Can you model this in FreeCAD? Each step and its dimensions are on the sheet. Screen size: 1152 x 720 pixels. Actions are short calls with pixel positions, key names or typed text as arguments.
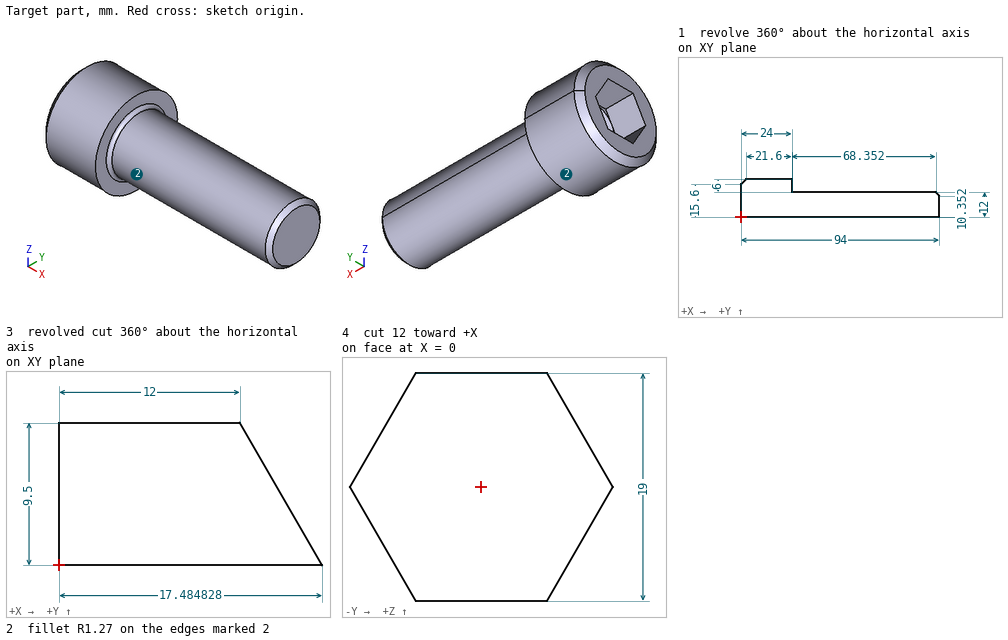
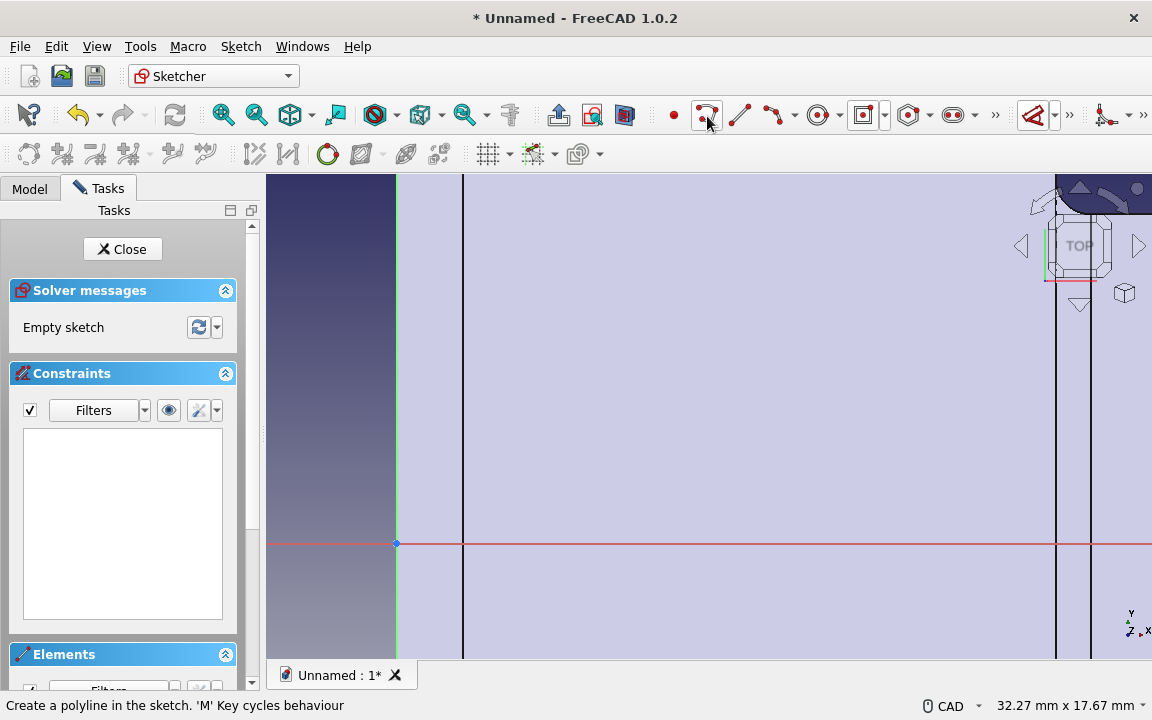
click(397, 544)
click(877, 535)
click(726, 283)
click(406, 283)
click(397, 544)
key(Escape)
key(Escape)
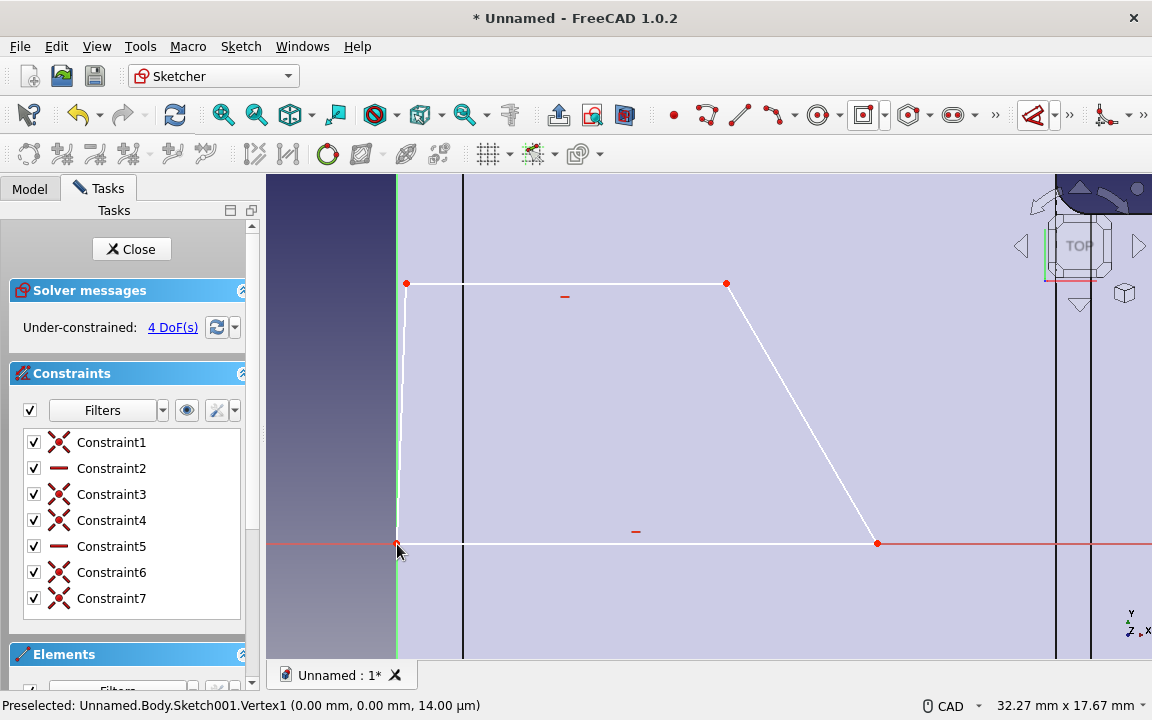
click(400, 466)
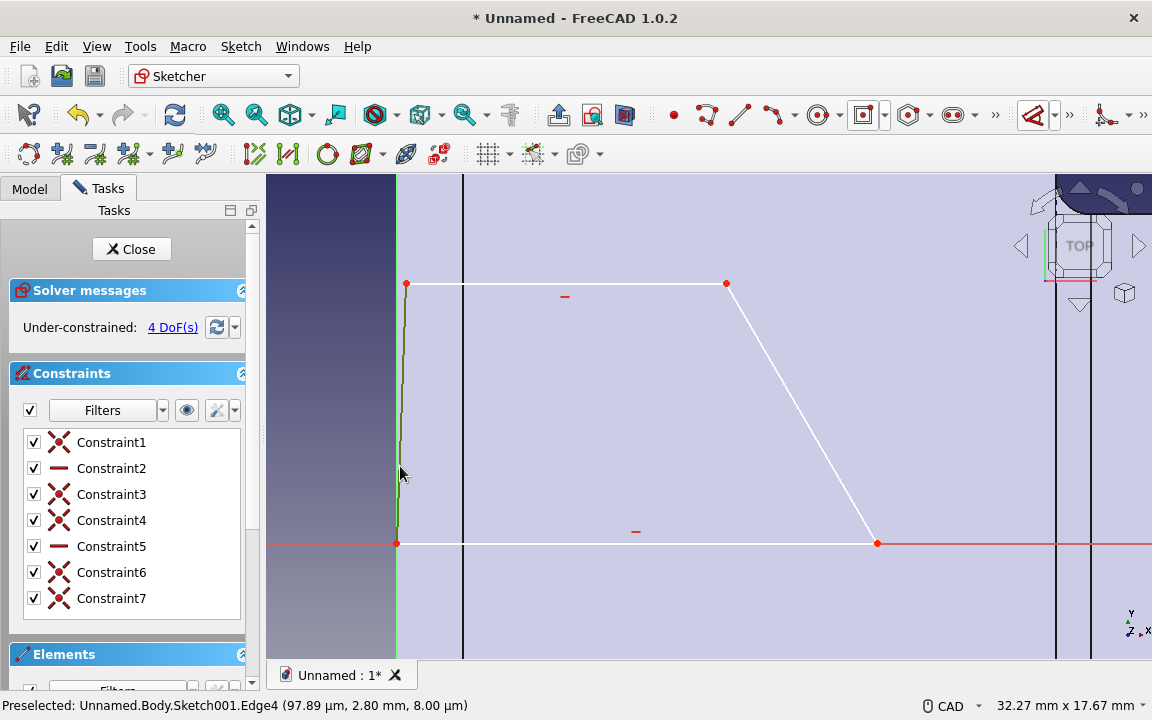
key(v)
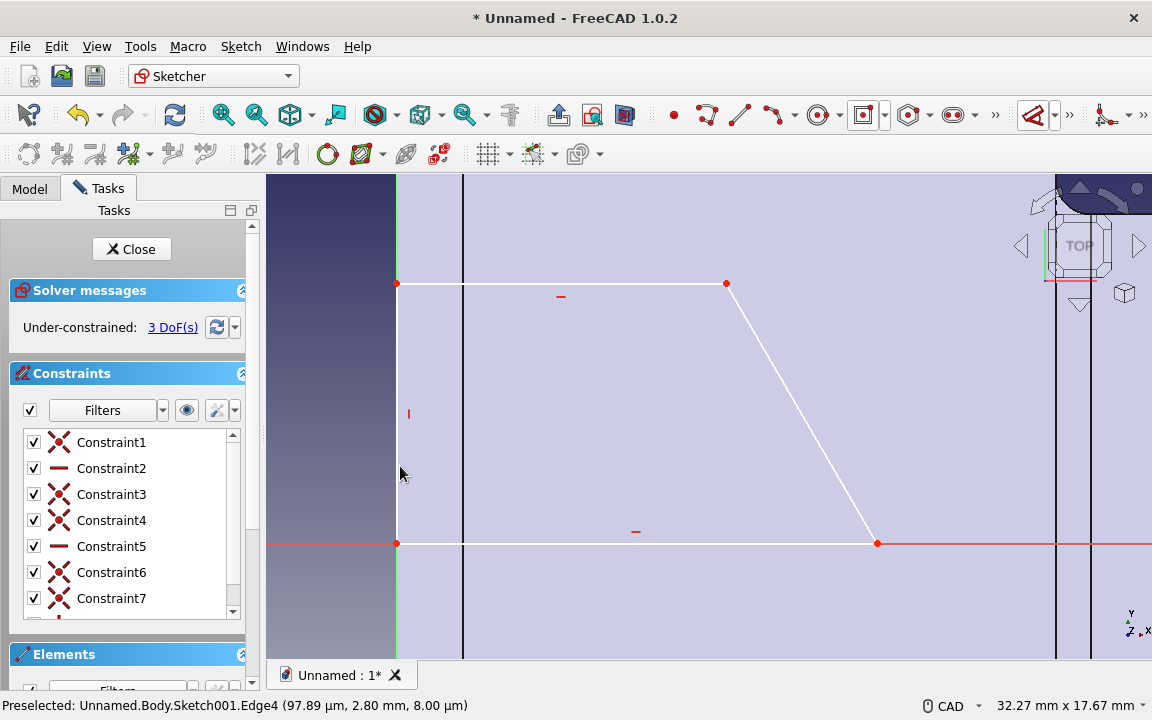
click(627, 284)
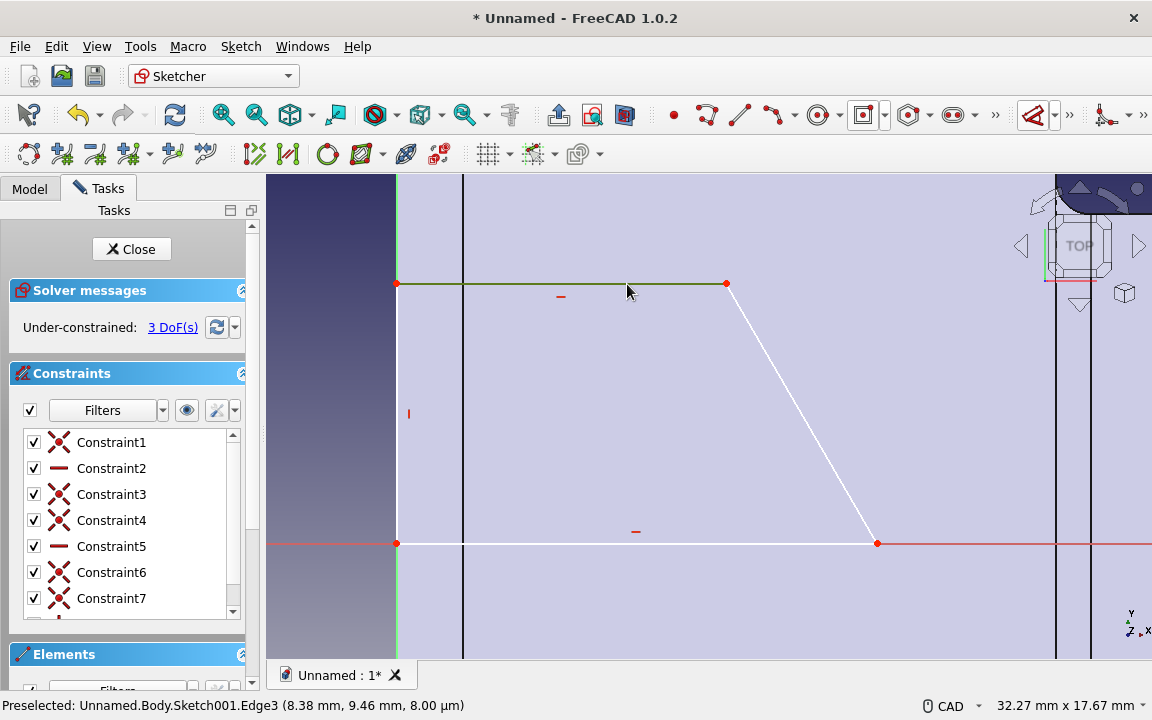
key(l)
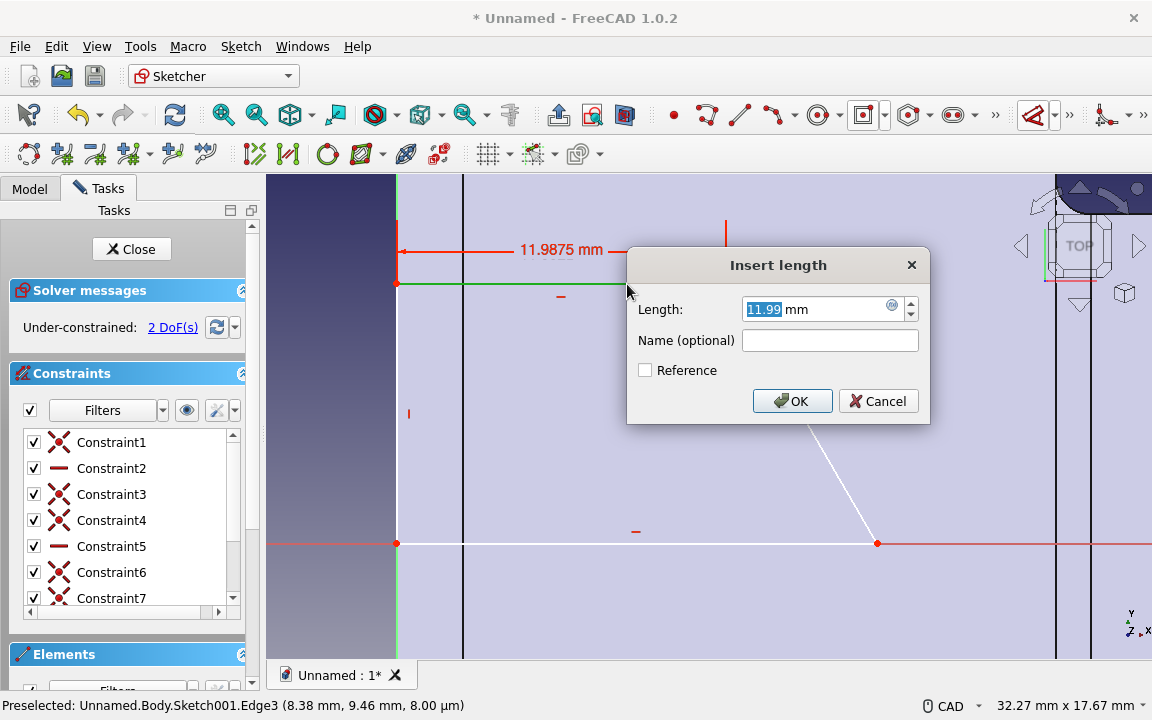
text(12)
key(Return)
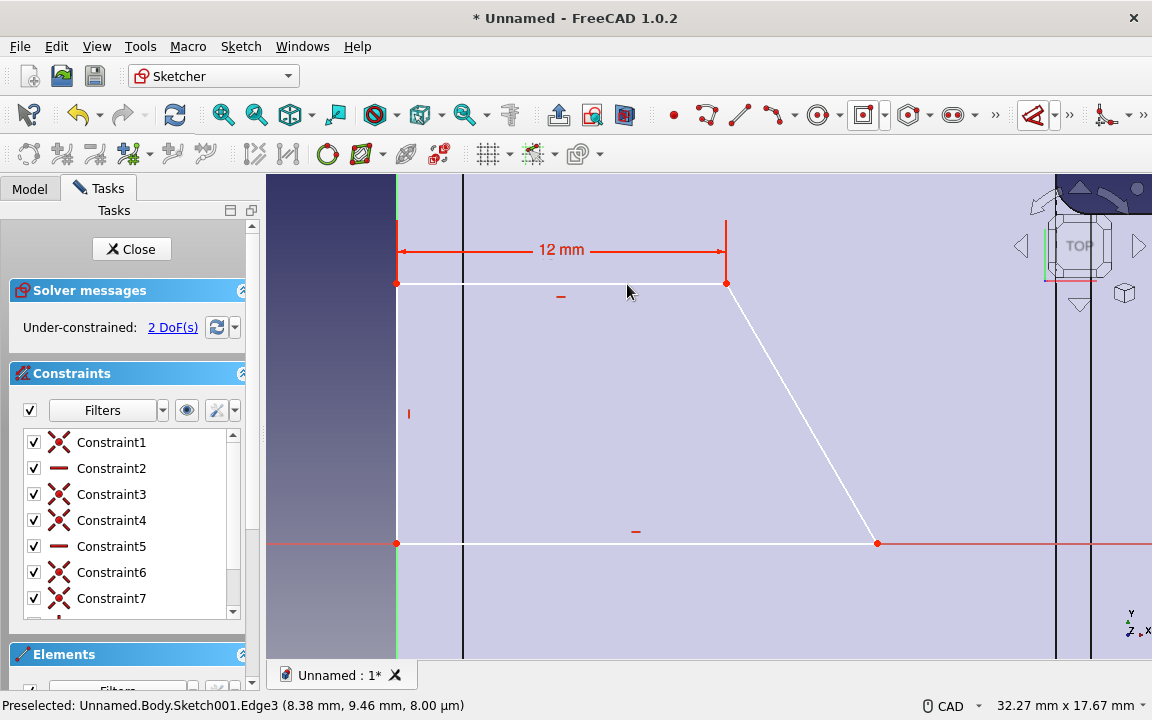
click(397, 362)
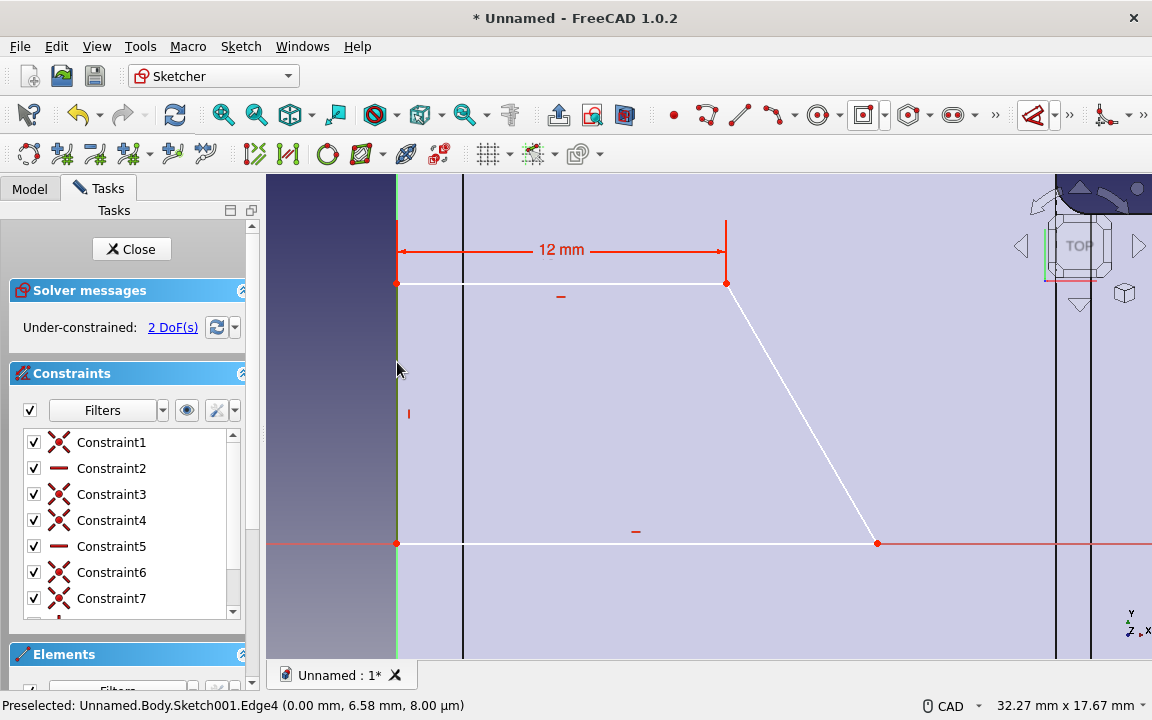
key(i)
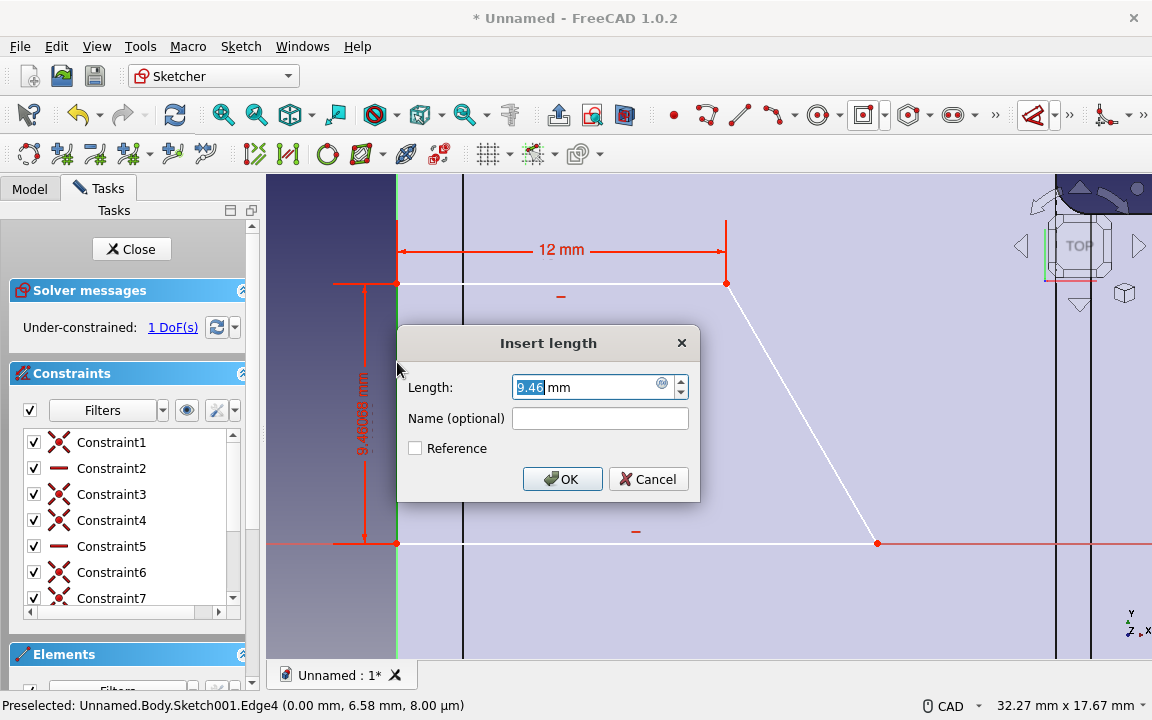
text(9.5)
key(Return)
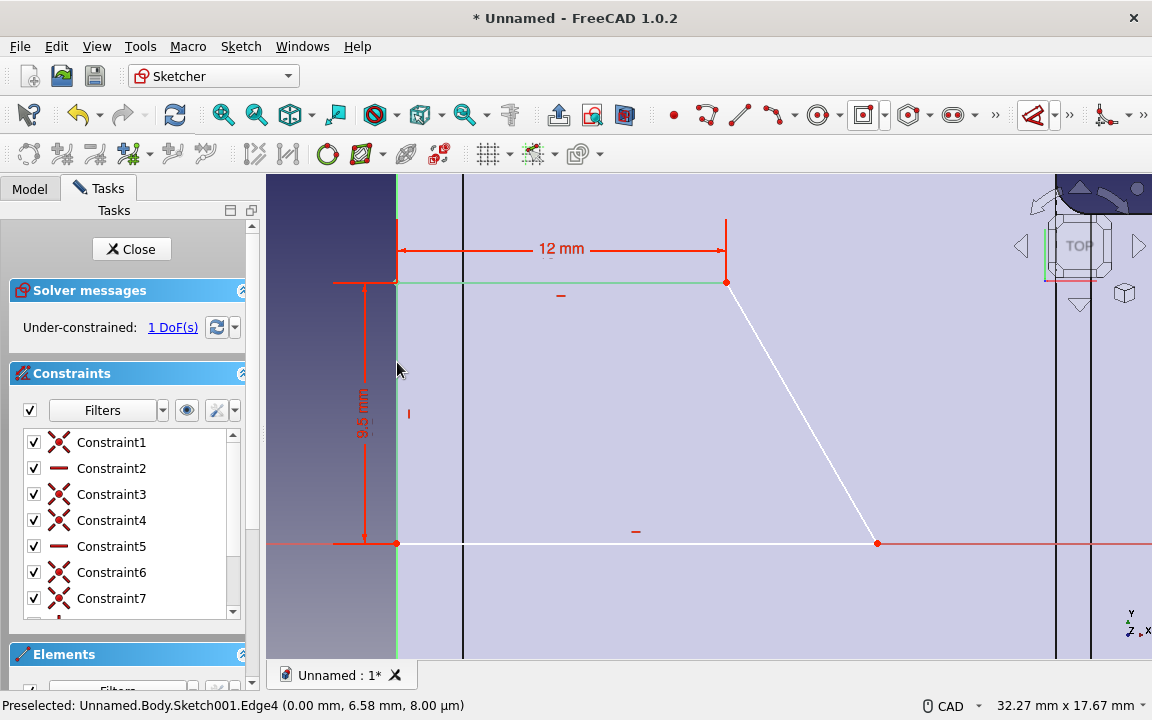
click(541, 544)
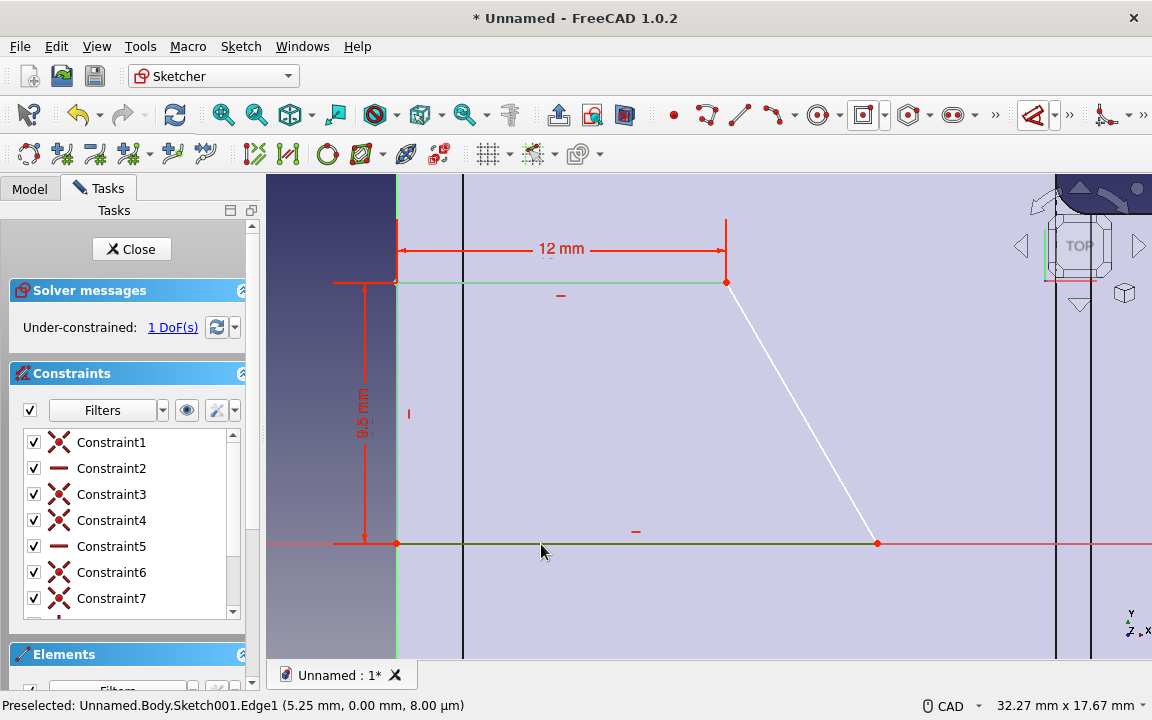
click(1054, 116)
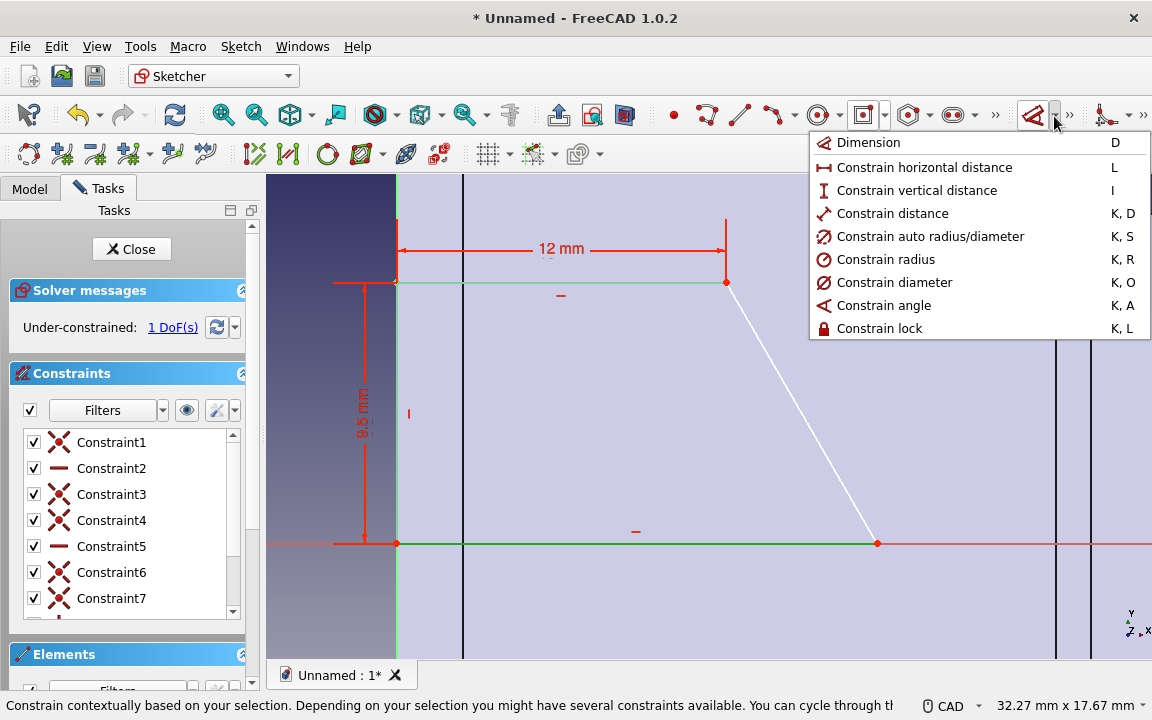
click(980, 168)